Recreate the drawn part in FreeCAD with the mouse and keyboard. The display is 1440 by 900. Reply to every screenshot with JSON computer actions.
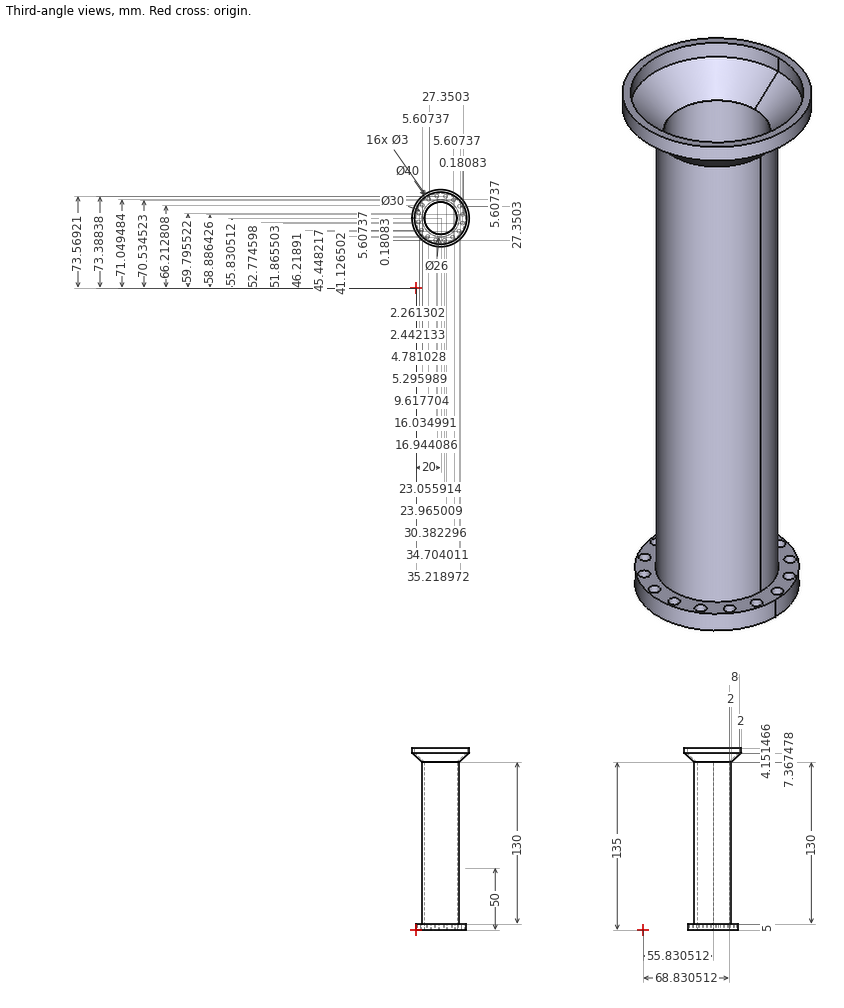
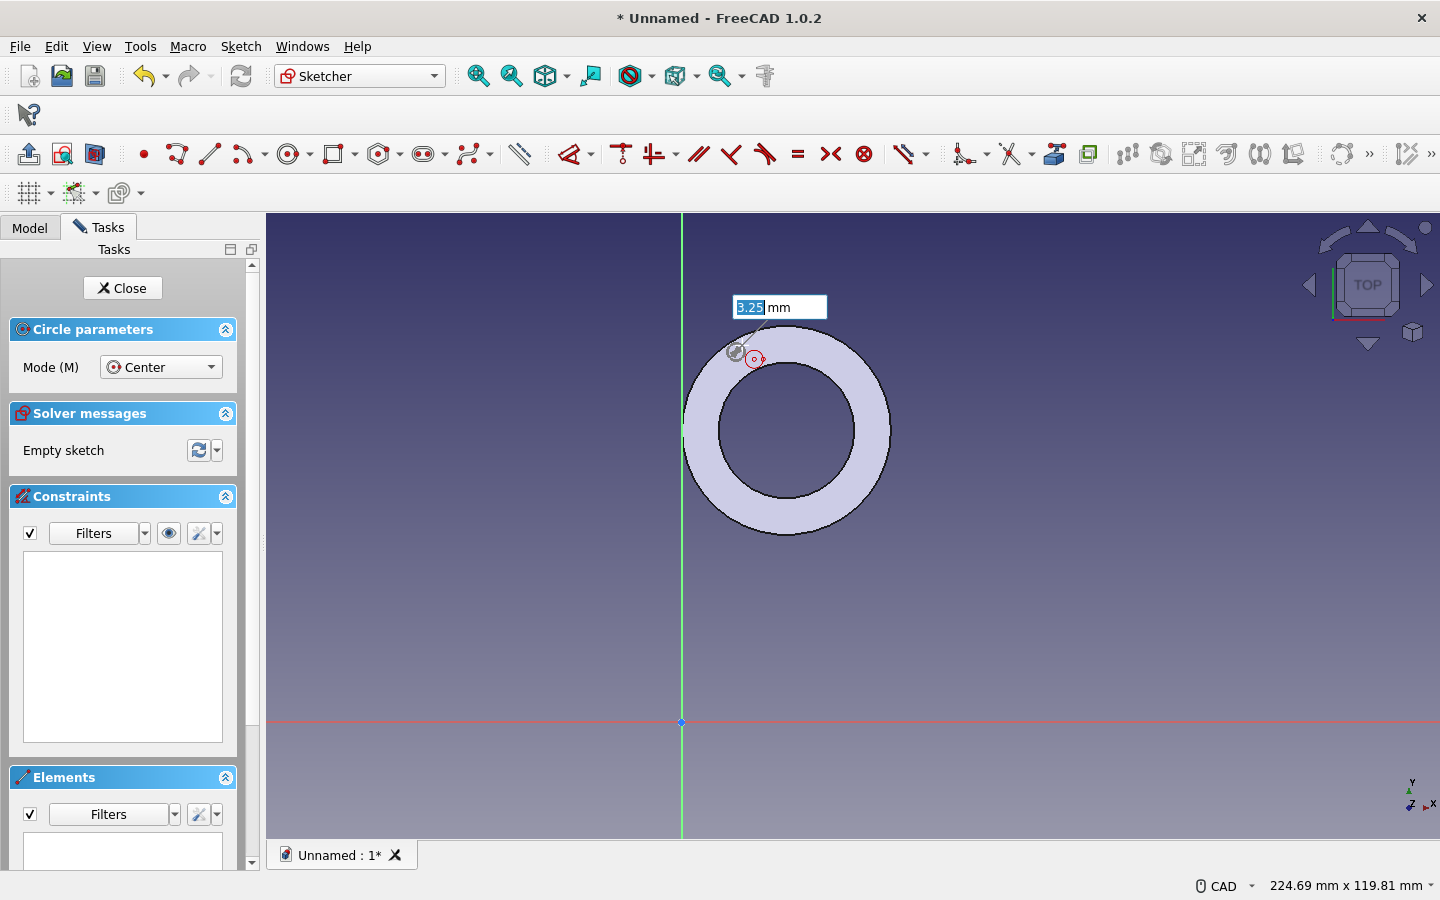
{"action": "type", "text": "3"}
{"action": "key", "text": "Return"}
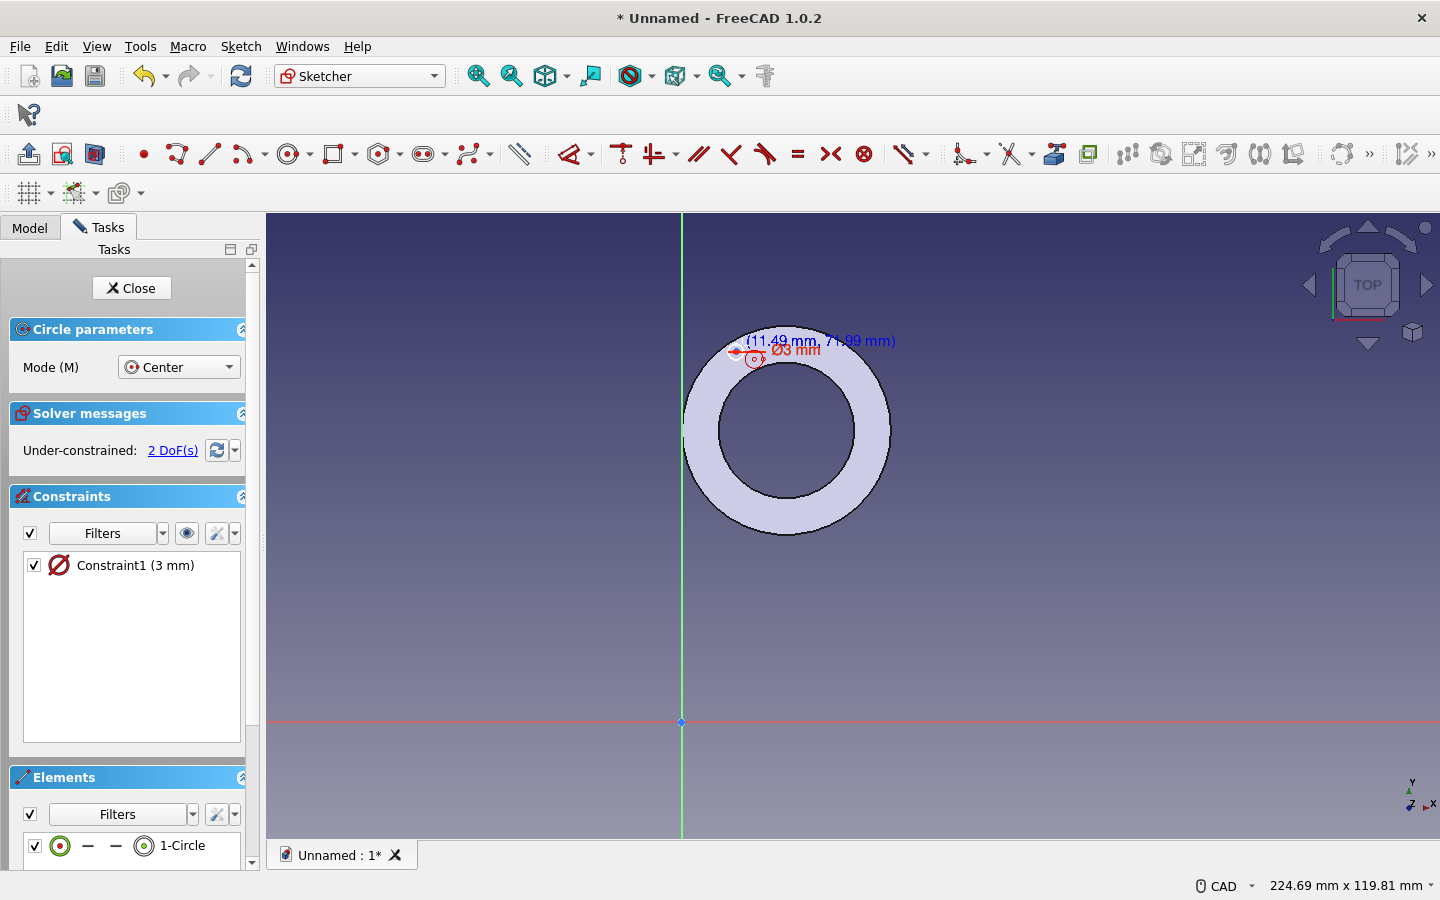
{"action": "scroll", "coordinate": [770, 338], "scroll_direction": "up", "scroll_amount": 6}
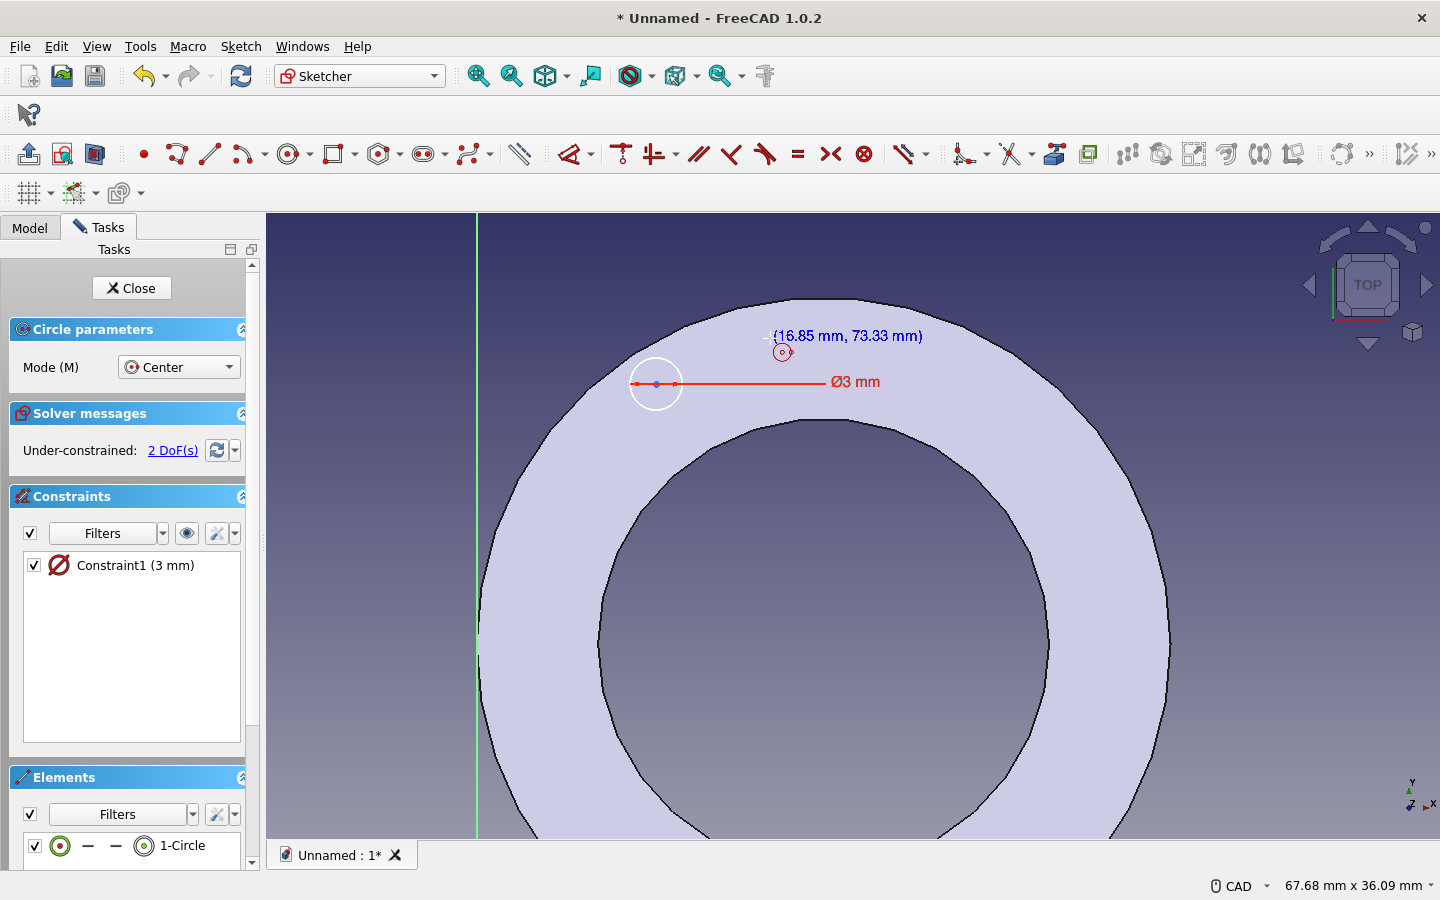
{"action": "scroll", "coordinate": [771, 338], "scroll_direction": "down", "scroll_amount": 6}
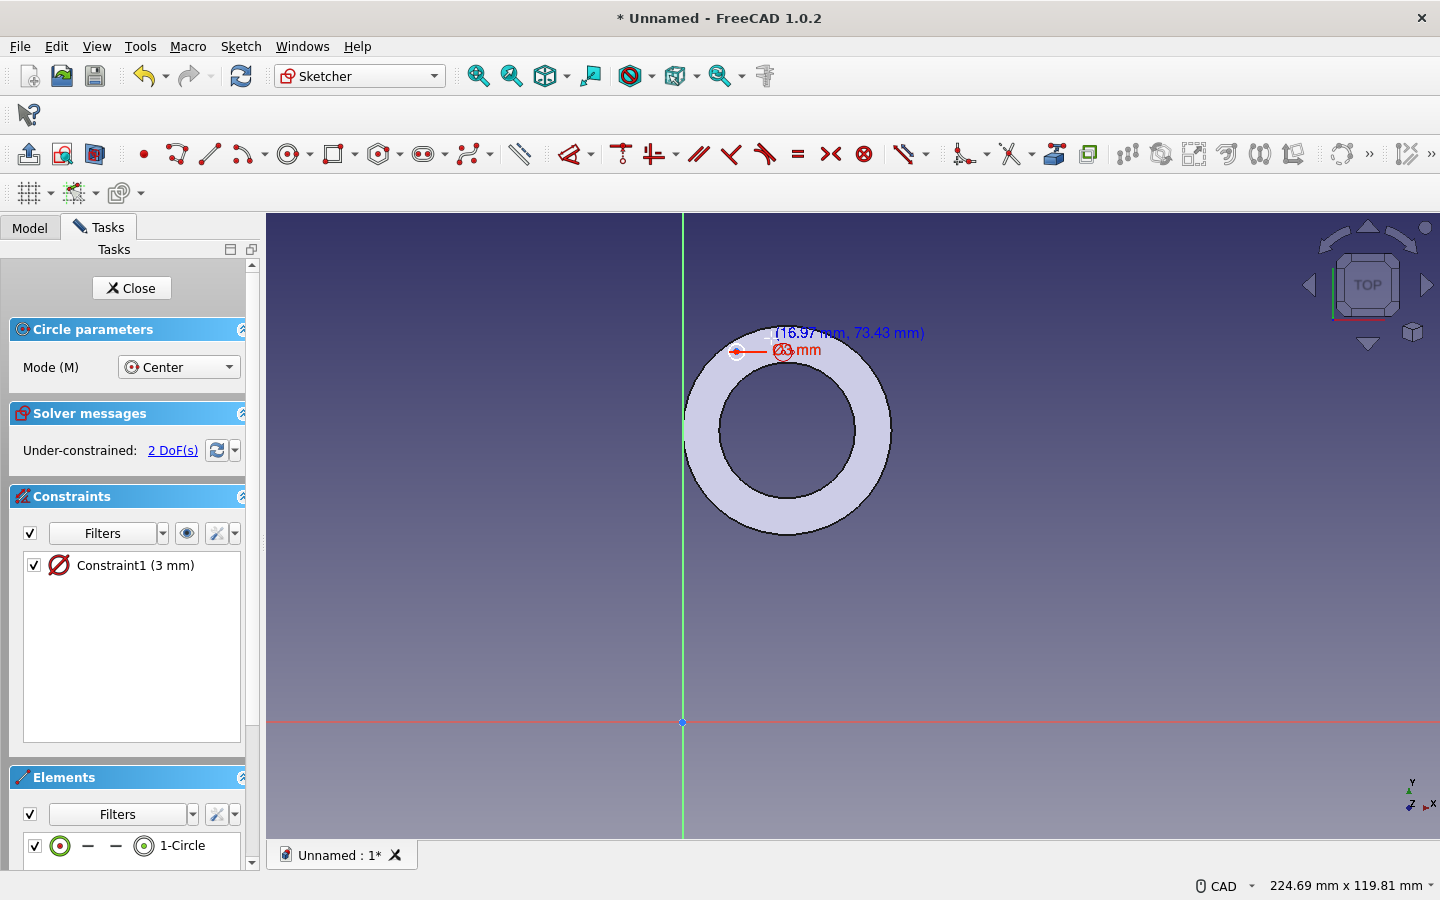
{"action": "left_click", "coordinate": [771, 338]}
{"action": "mouse_move", "coordinate": [777, 332]}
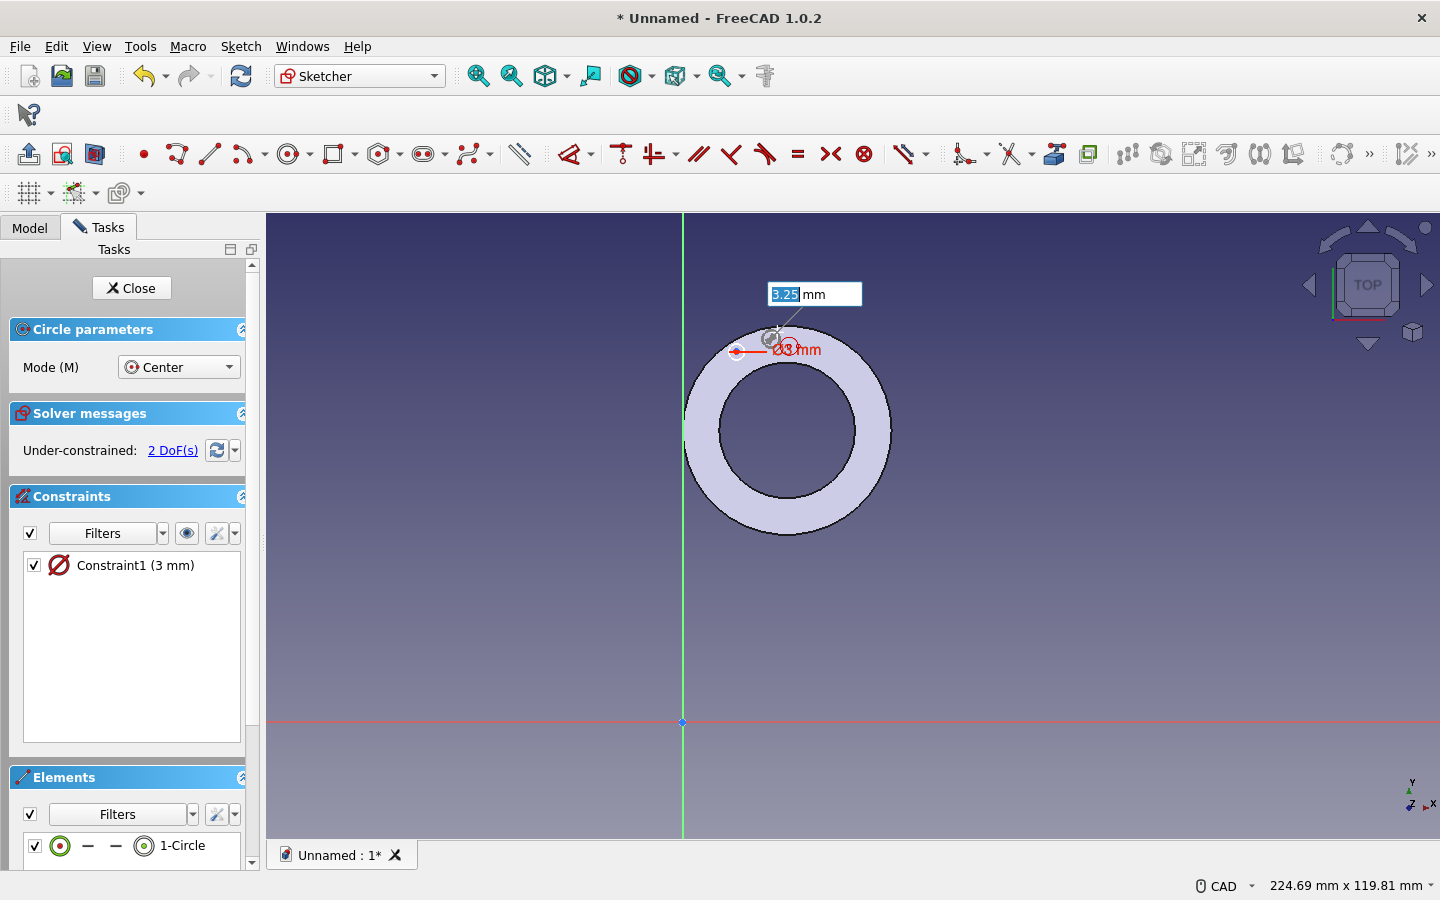
{"action": "type", "text": "3"}
{"action": "key", "text": "Return"}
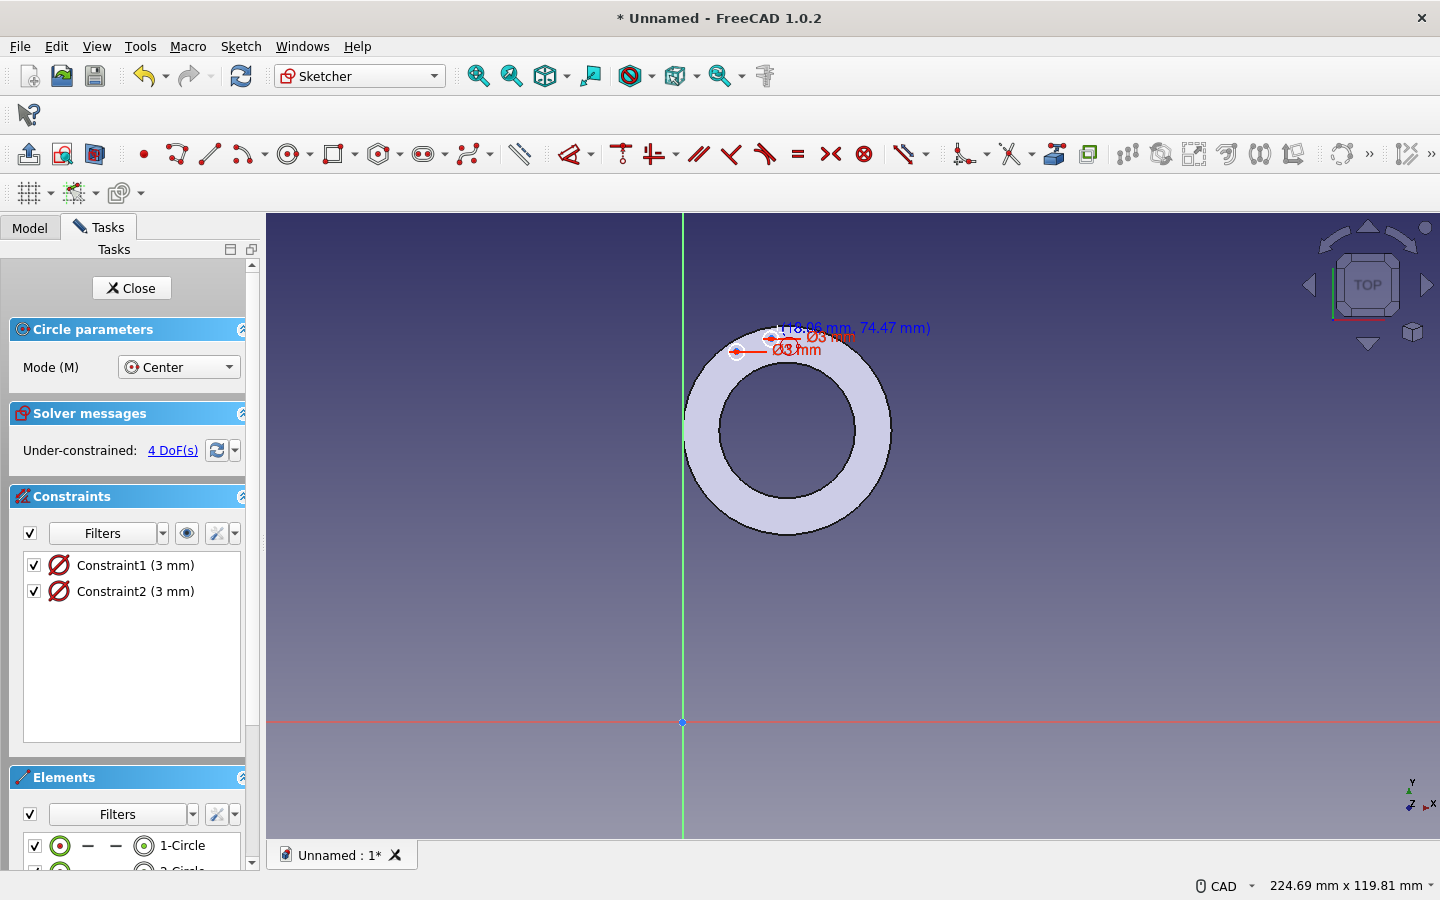
{"action": "scroll", "coordinate": [808, 339], "scroll_direction": "up", "scroll_amount": 6}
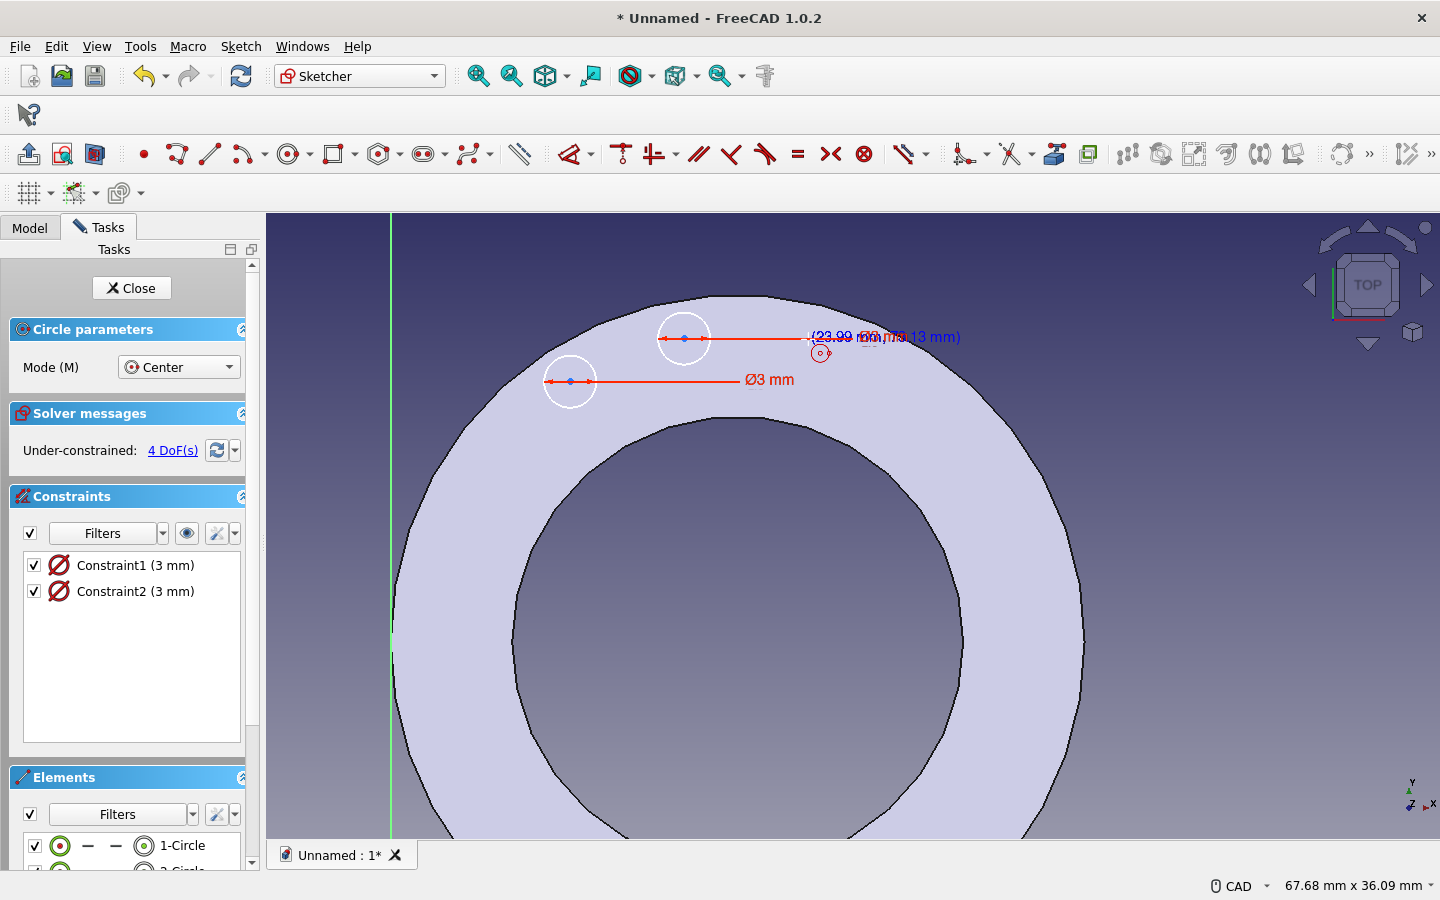
{"action": "scroll", "coordinate": [808, 339], "scroll_direction": "down", "scroll_amount": 6}